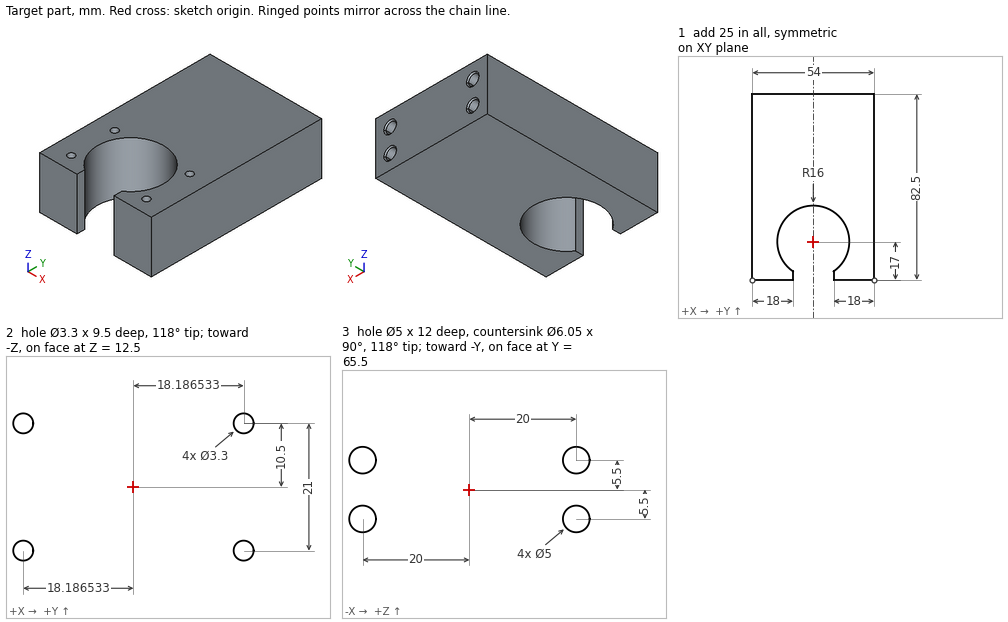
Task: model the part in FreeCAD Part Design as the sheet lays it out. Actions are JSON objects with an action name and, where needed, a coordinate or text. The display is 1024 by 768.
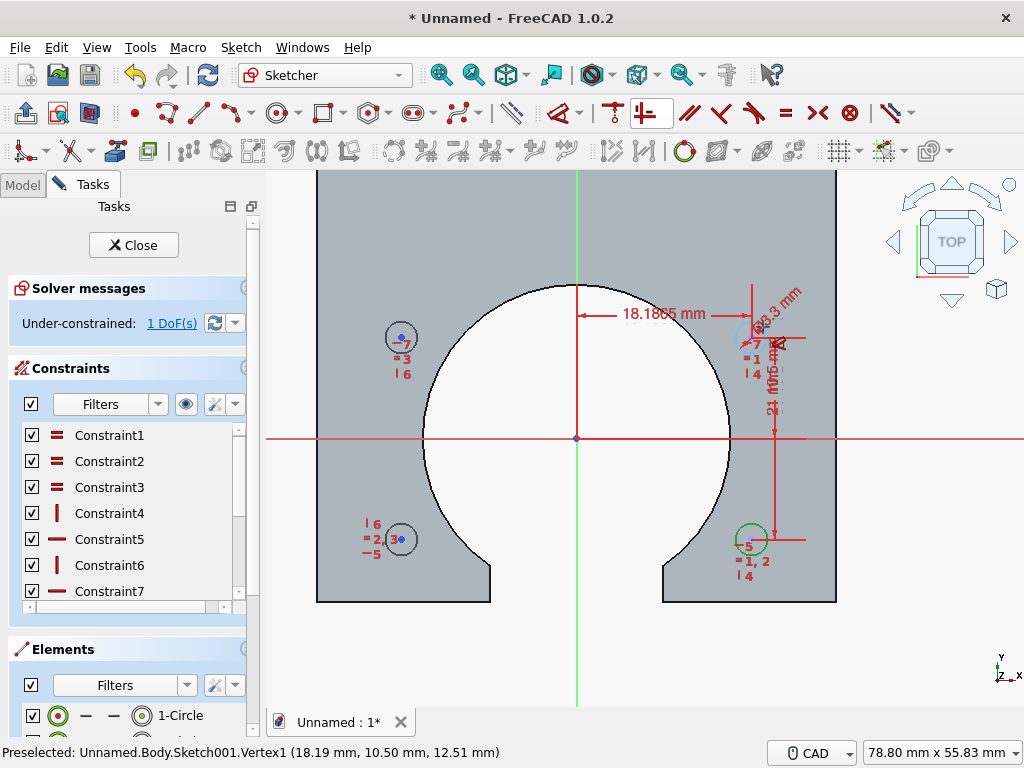
{"action": "left_click", "coordinate": [401, 540]}
{"action": "left_click", "coordinate": [489, 574]}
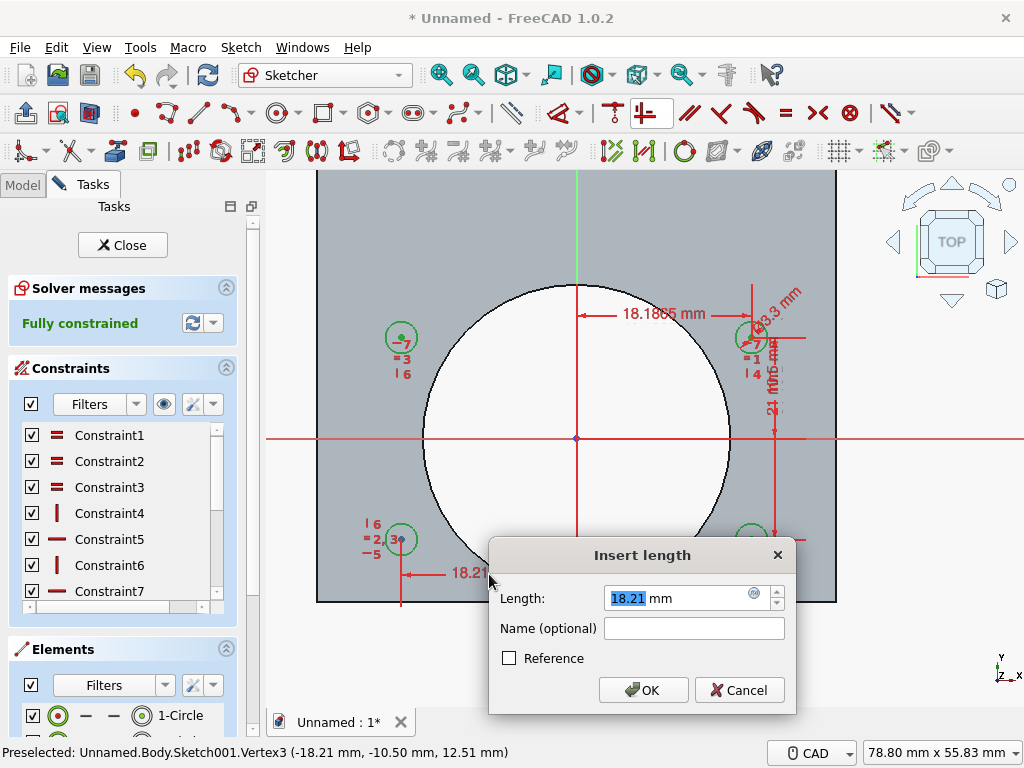
{"action": "type", "text": "18.186533"}
{"action": "key", "text": "Return"}
{"action": "key", "text": "Escape"}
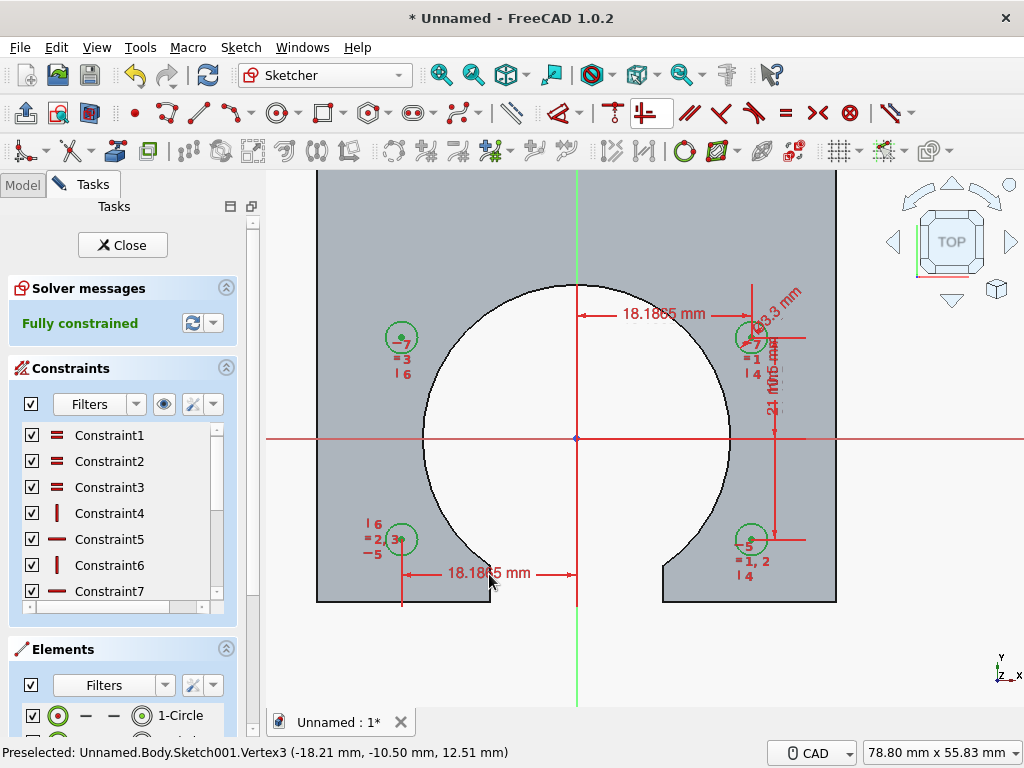
{"action": "left_click", "coordinate": [123, 245]}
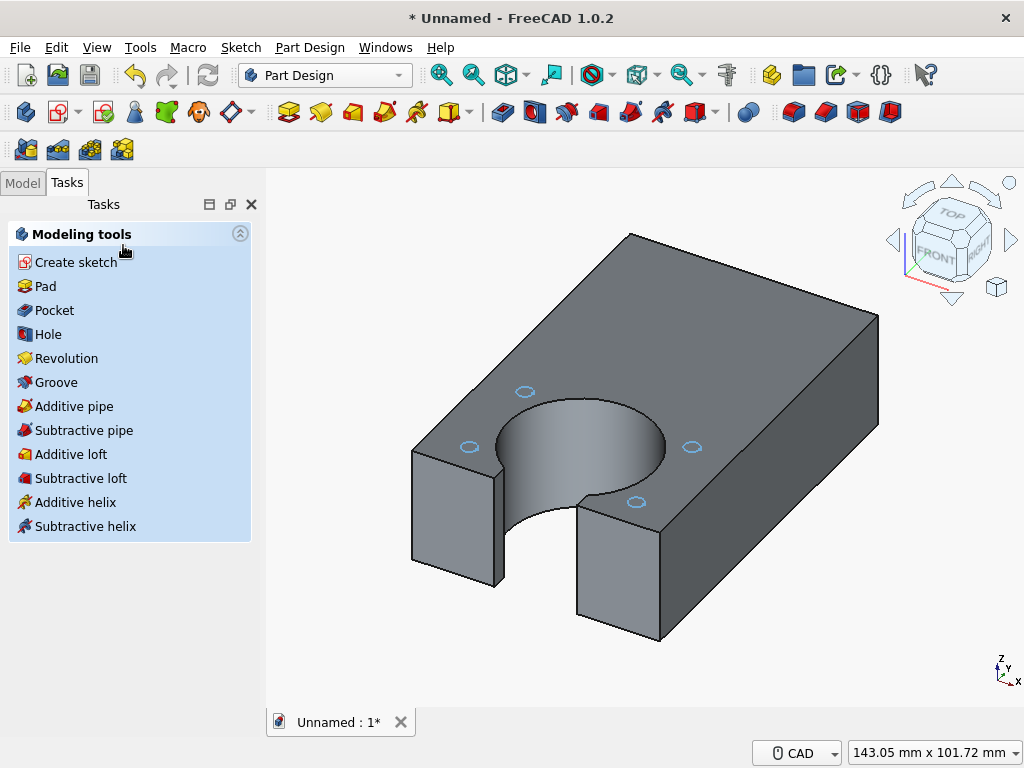
{"action": "left_click", "coordinate": [536, 112]}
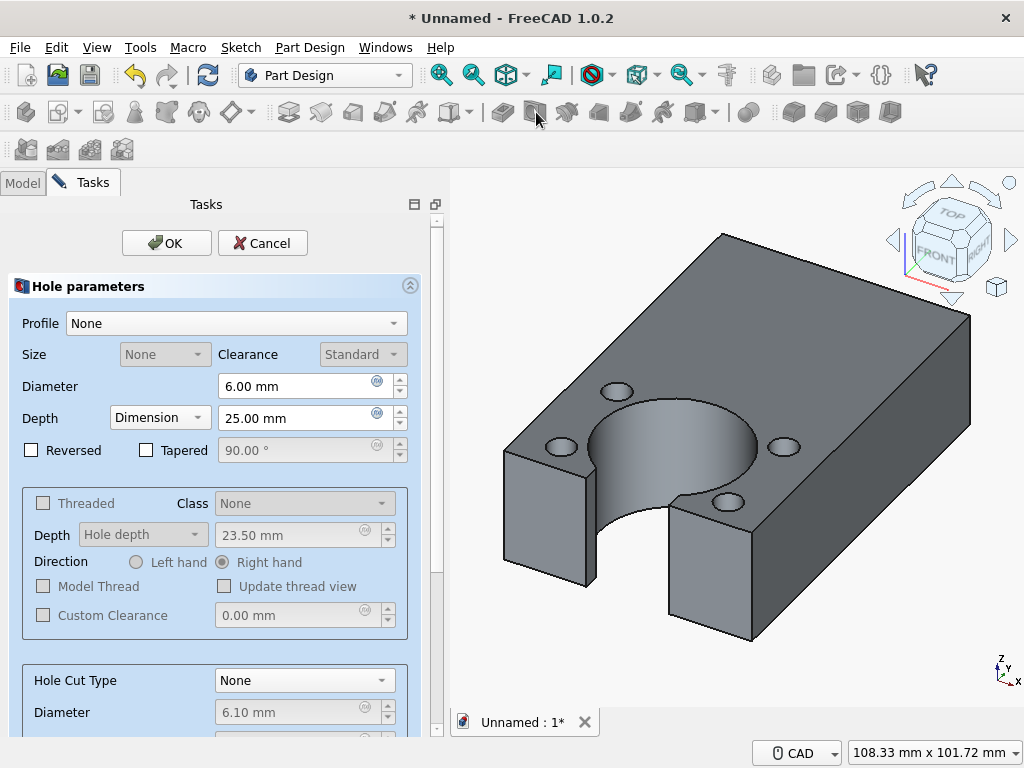
{"action": "triple_click", "coordinate": [305, 386]}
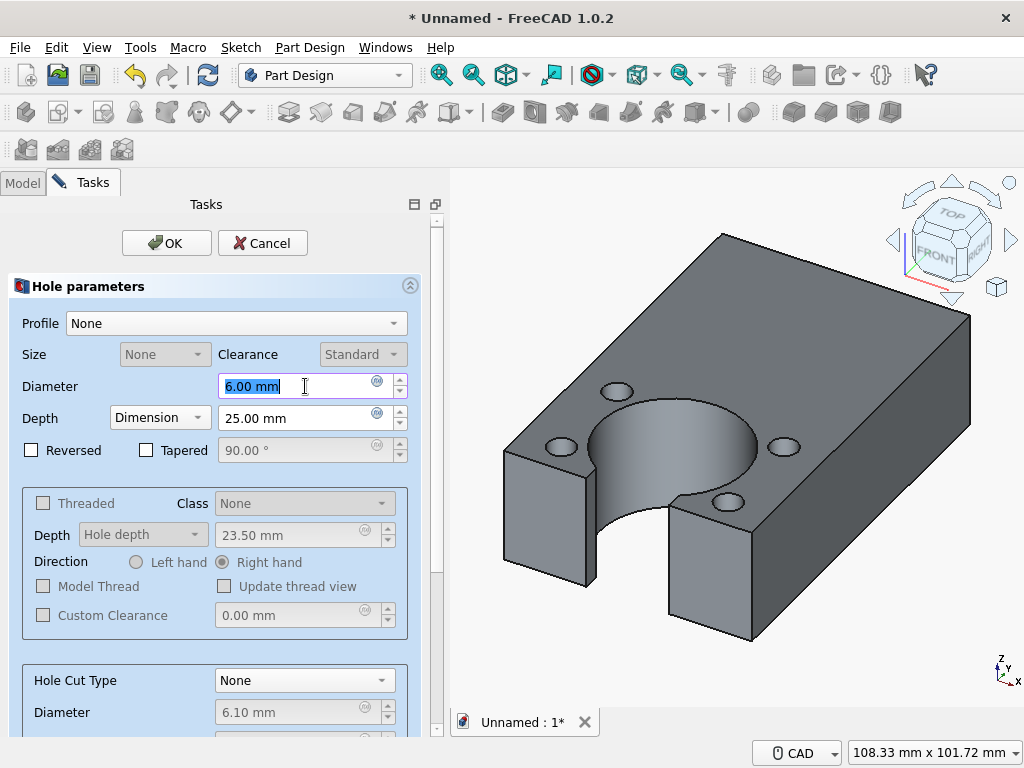
{"action": "type", "text": "3.3"}
{"action": "key", "text": "Tab"}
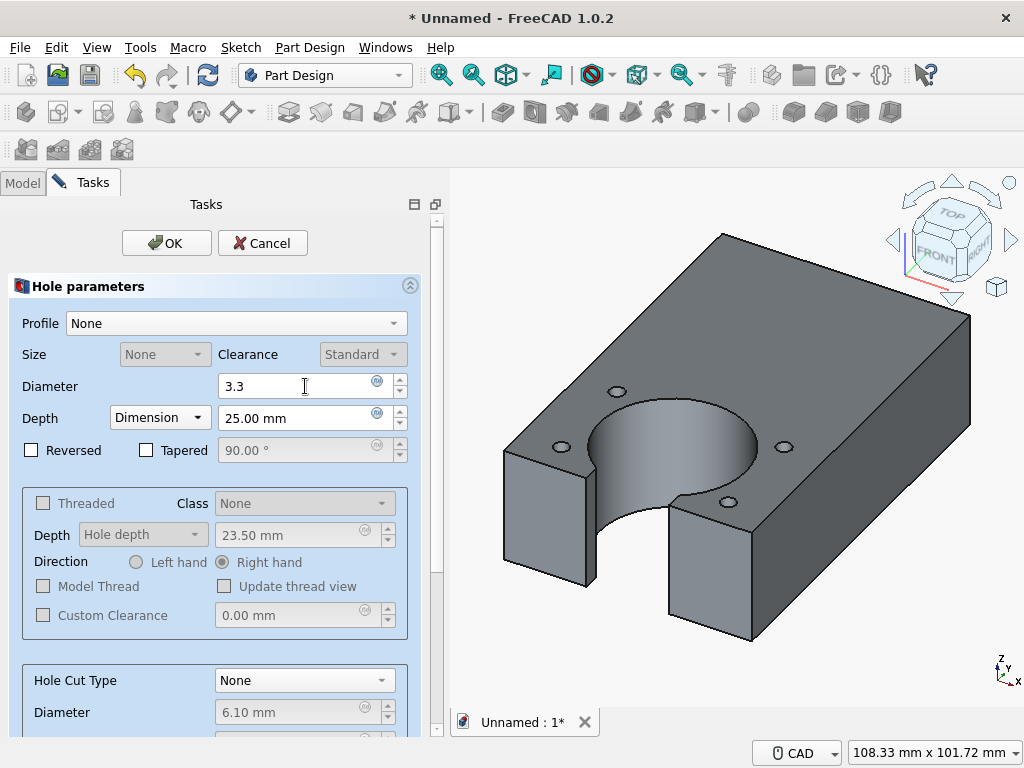
{"action": "triple_click", "coordinate": [305, 418]}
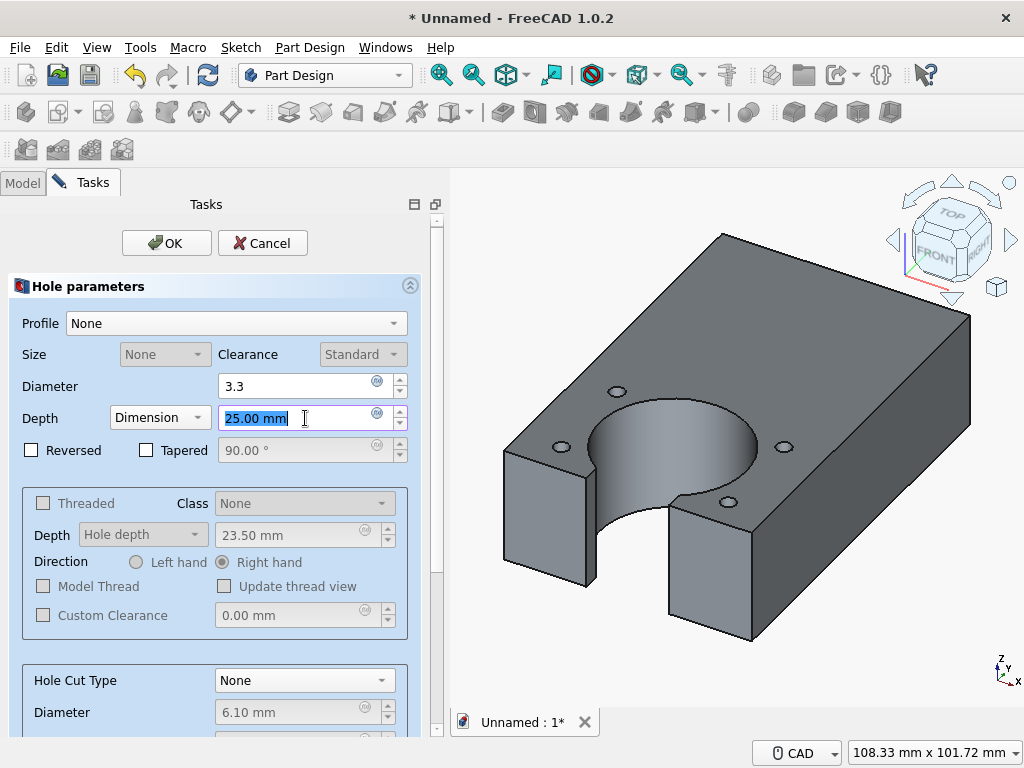
{"action": "type", "text": "9.5"}
{"action": "key", "text": "Tab"}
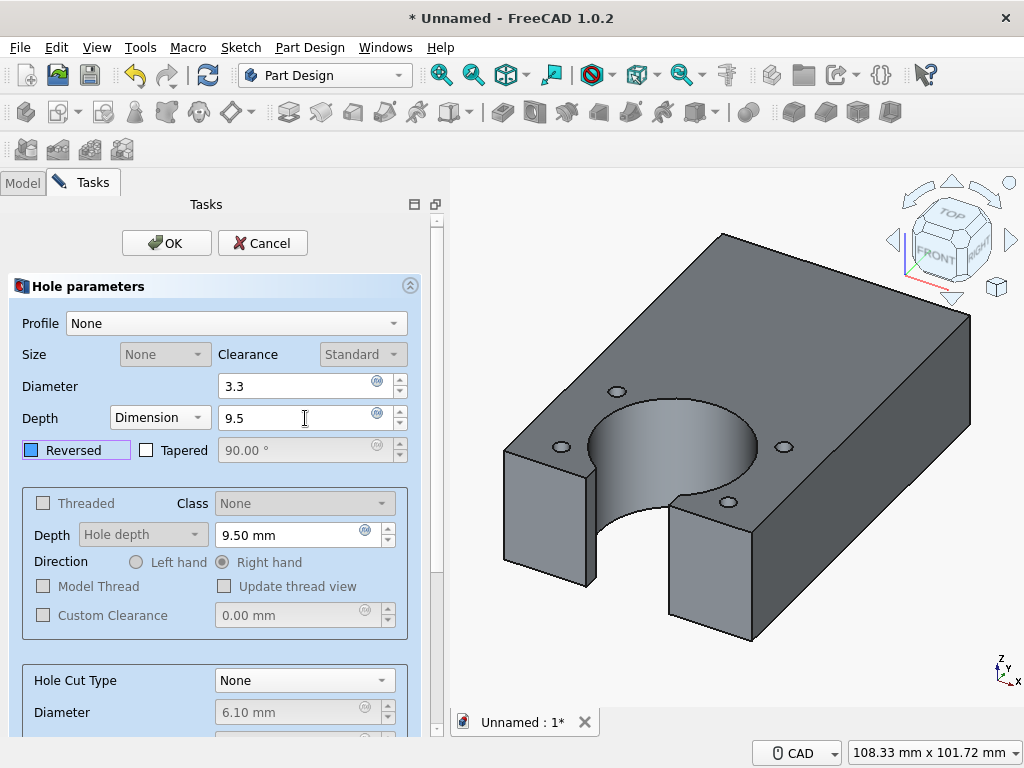
{"action": "left_click", "coordinate": [167, 243]}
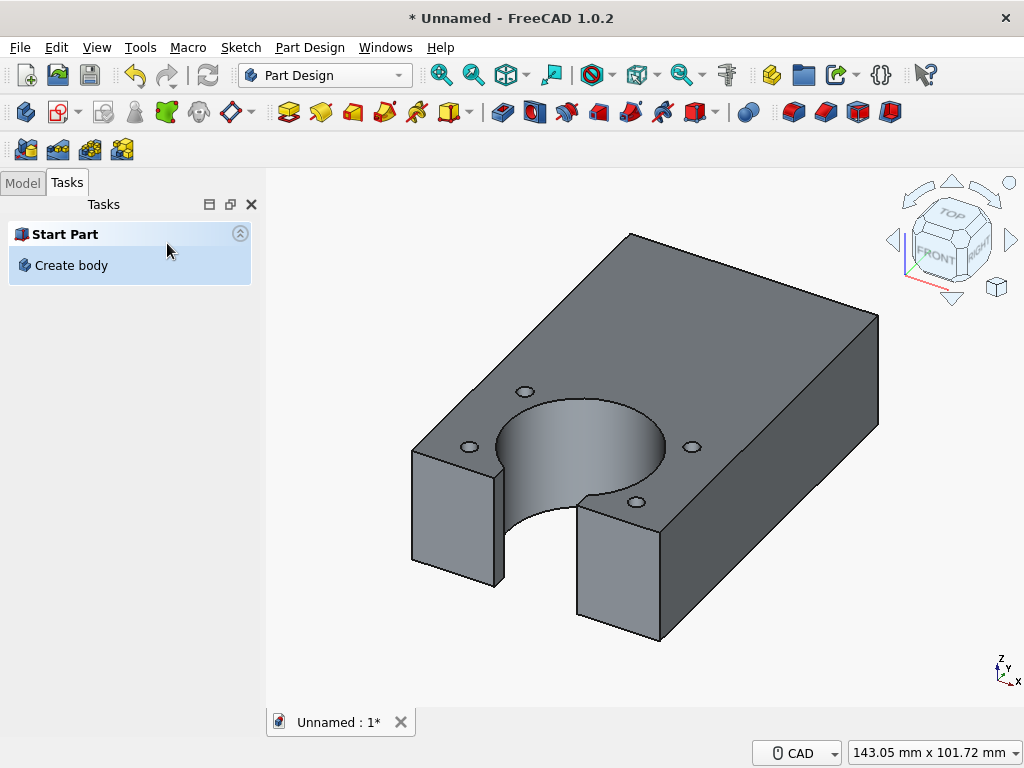
{"action": "key", "text": "4"}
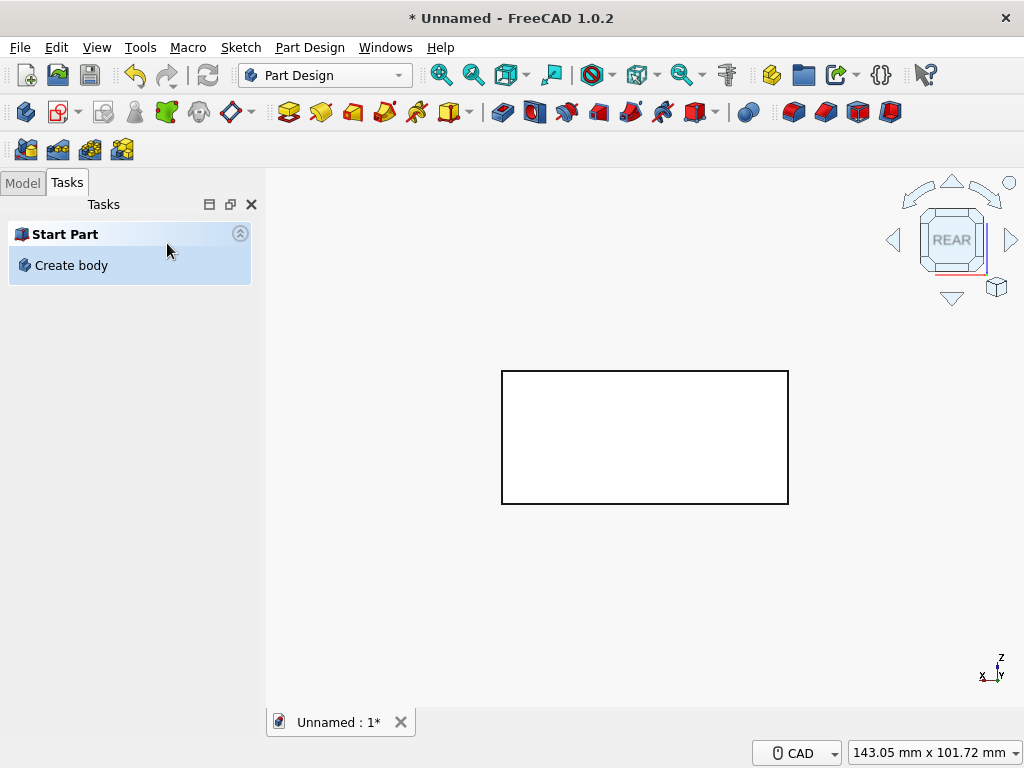
{"action": "key", "text": "v f"}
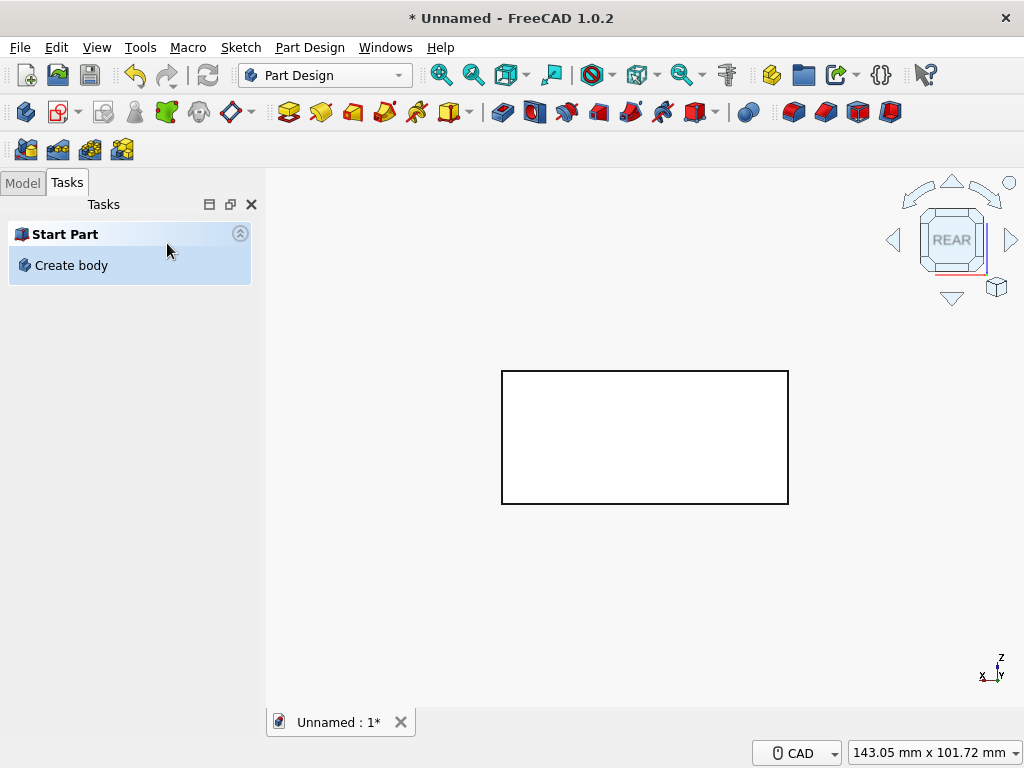
{"action": "left_click", "coordinate": [604, 437]}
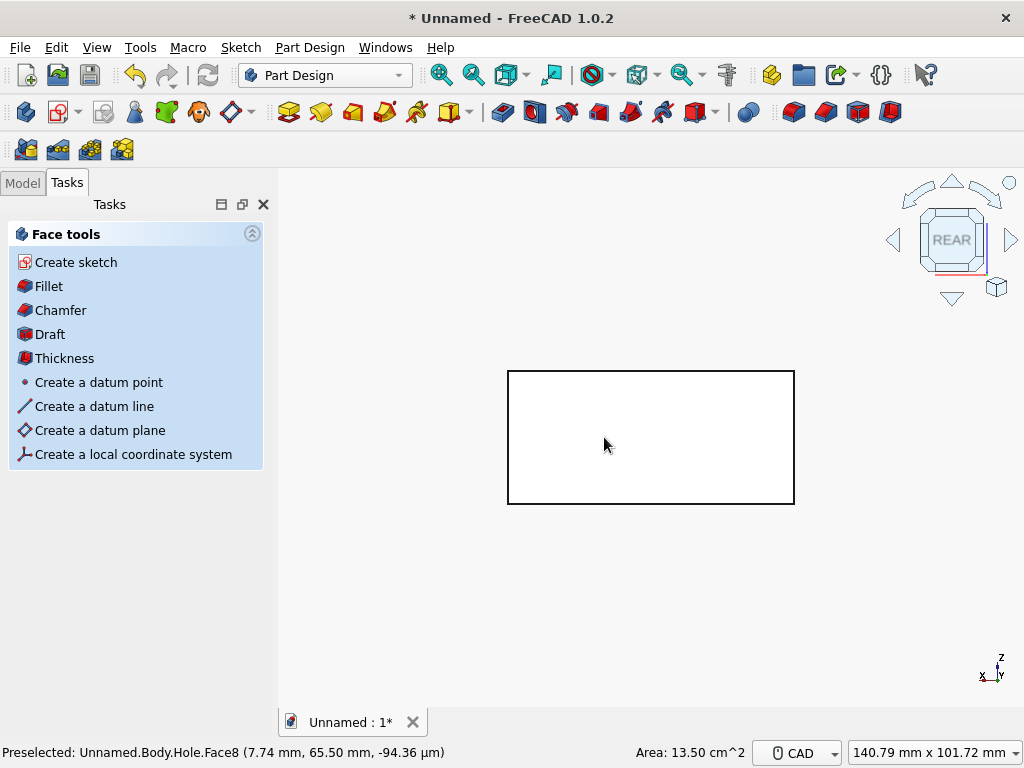
{"action": "left_click", "coordinate": [58, 112]}